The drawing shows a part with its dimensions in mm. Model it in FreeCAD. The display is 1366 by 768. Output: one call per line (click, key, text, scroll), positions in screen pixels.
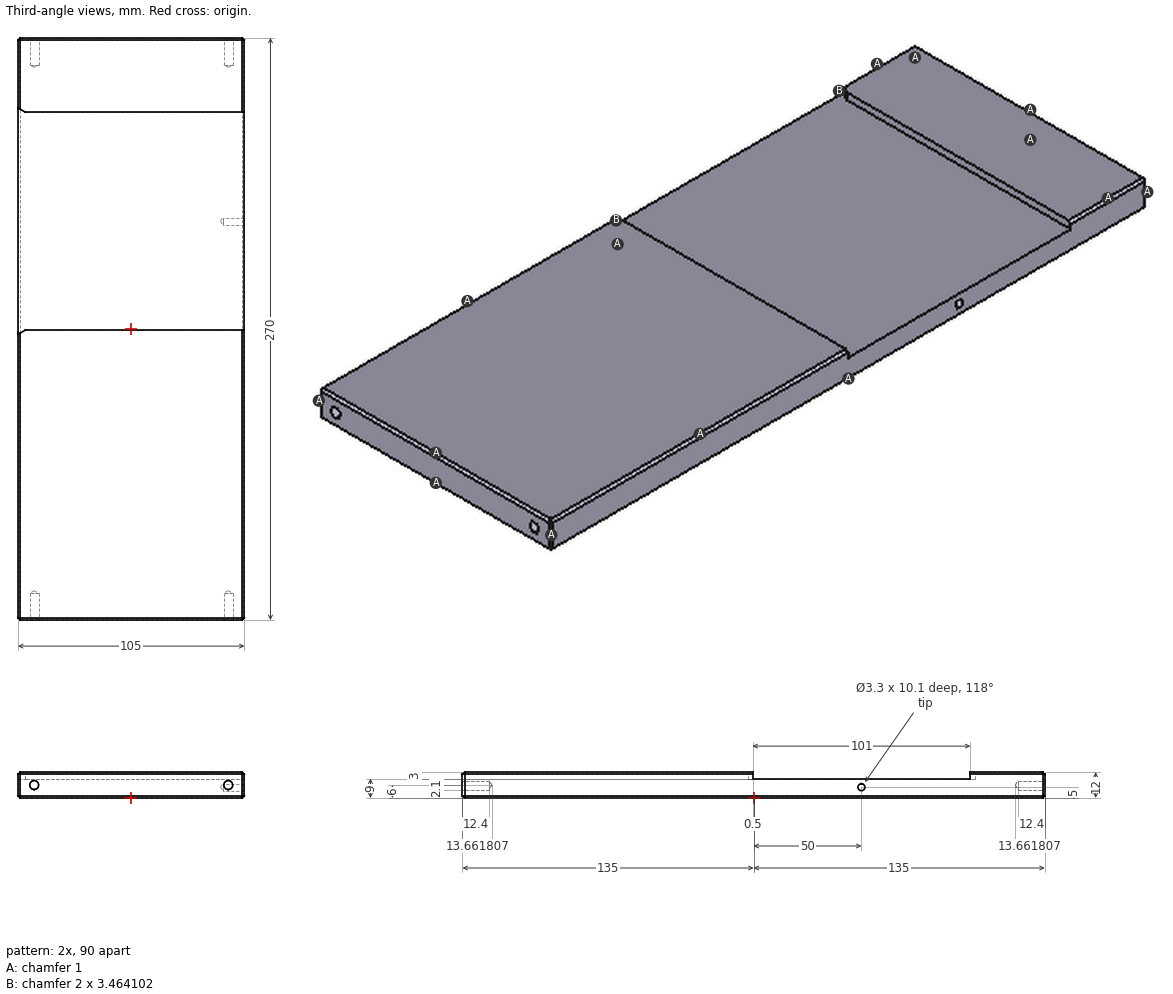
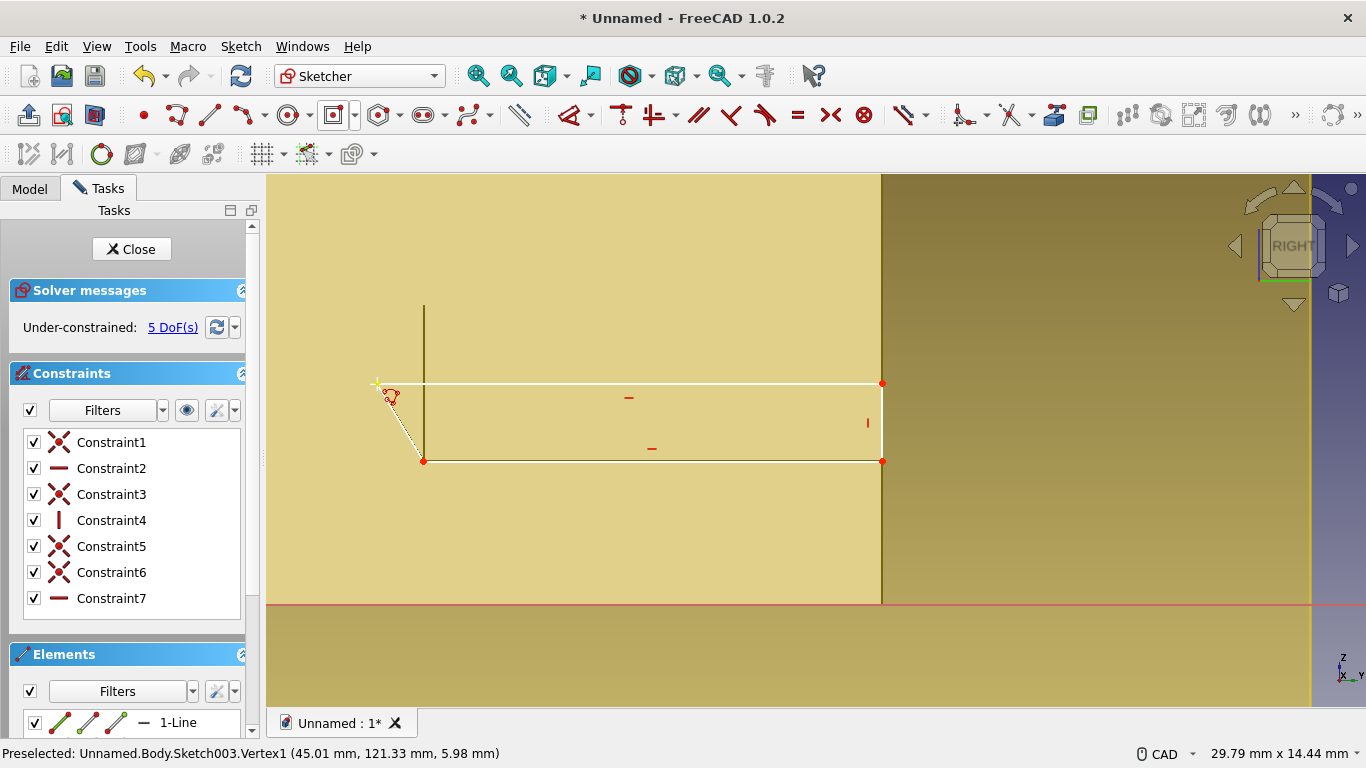
click(210, 116)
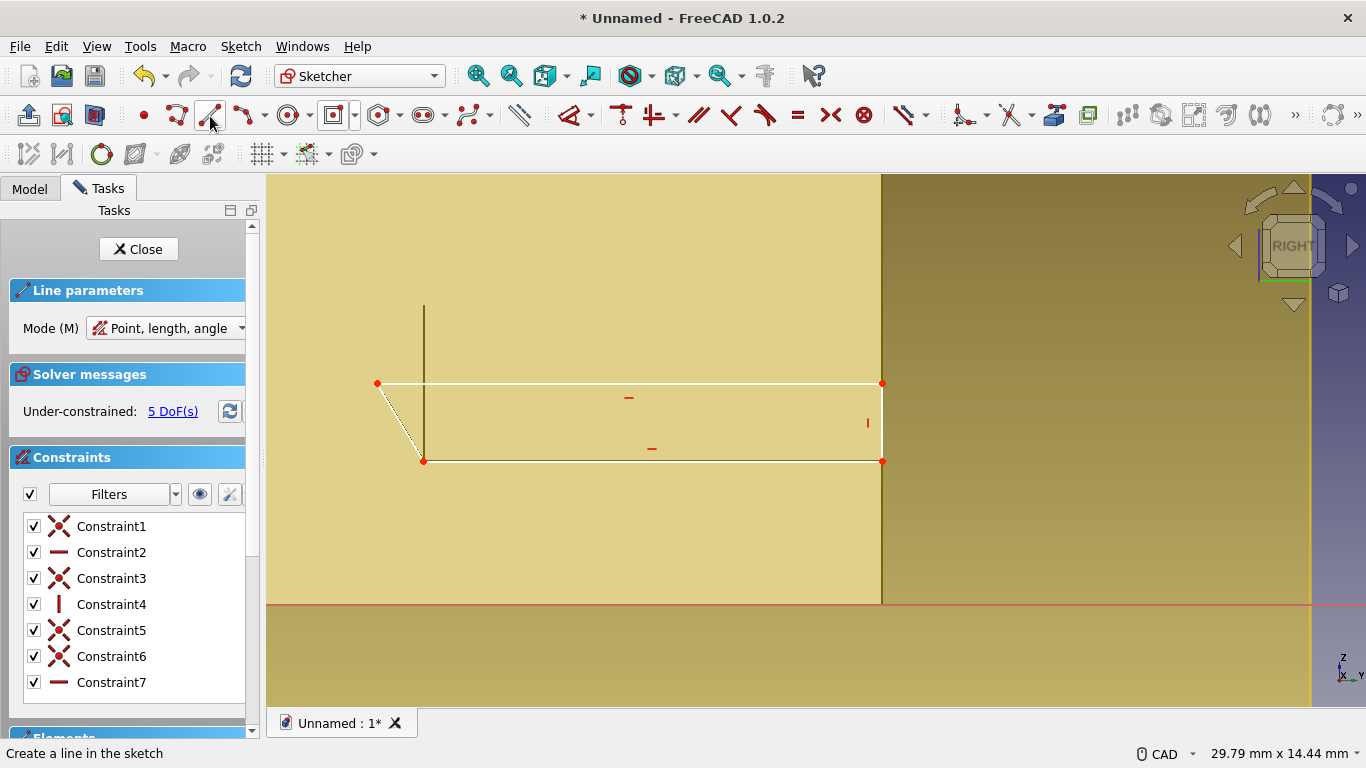
click(932, 383)
click(1083, 383)
key(Escape)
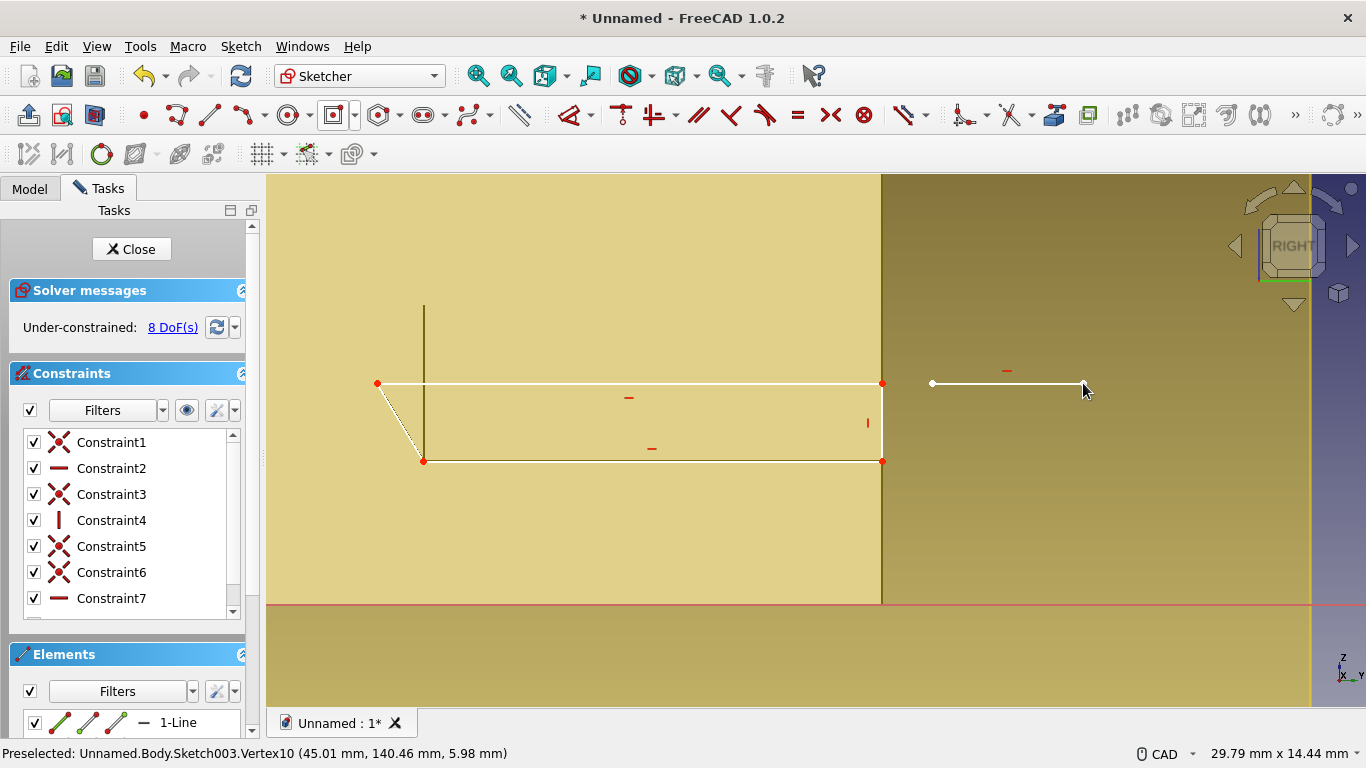
click(977, 384)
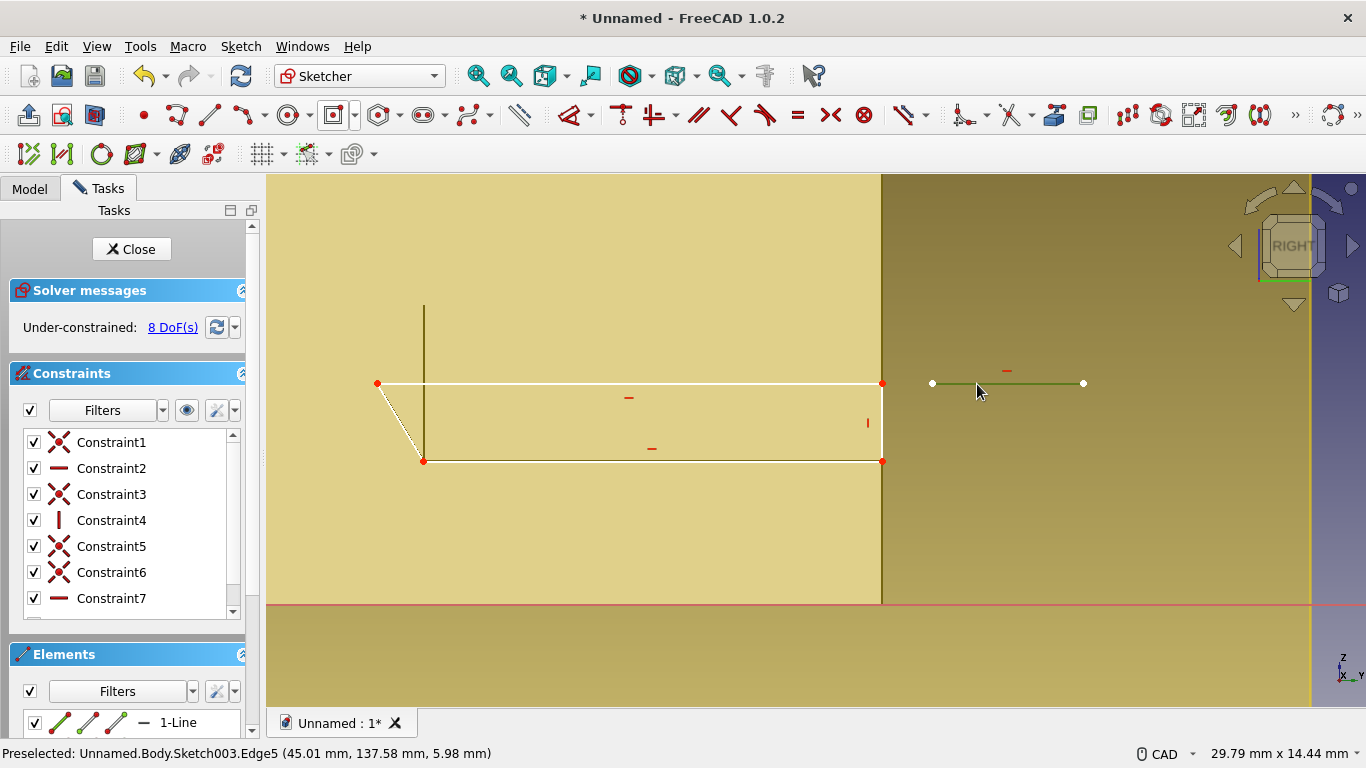
click(520, 116)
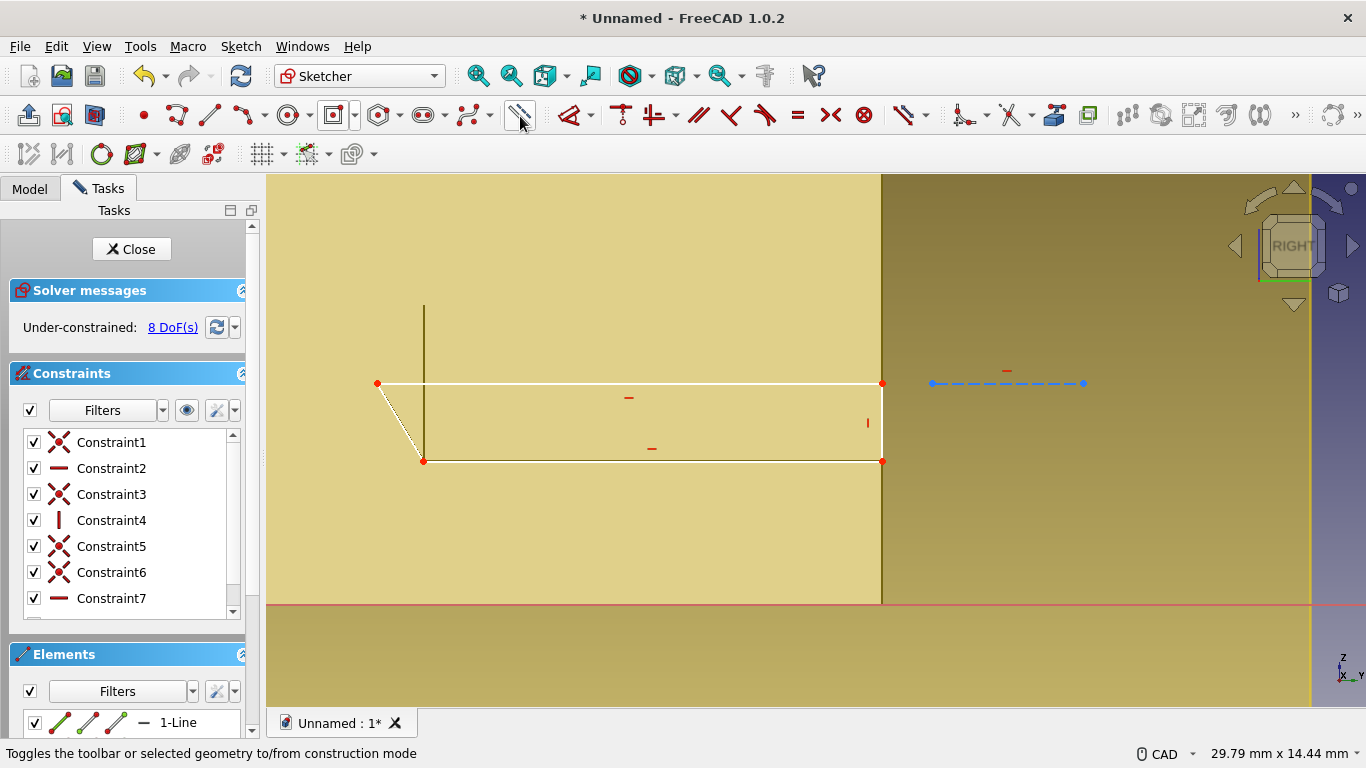
click(568, 116)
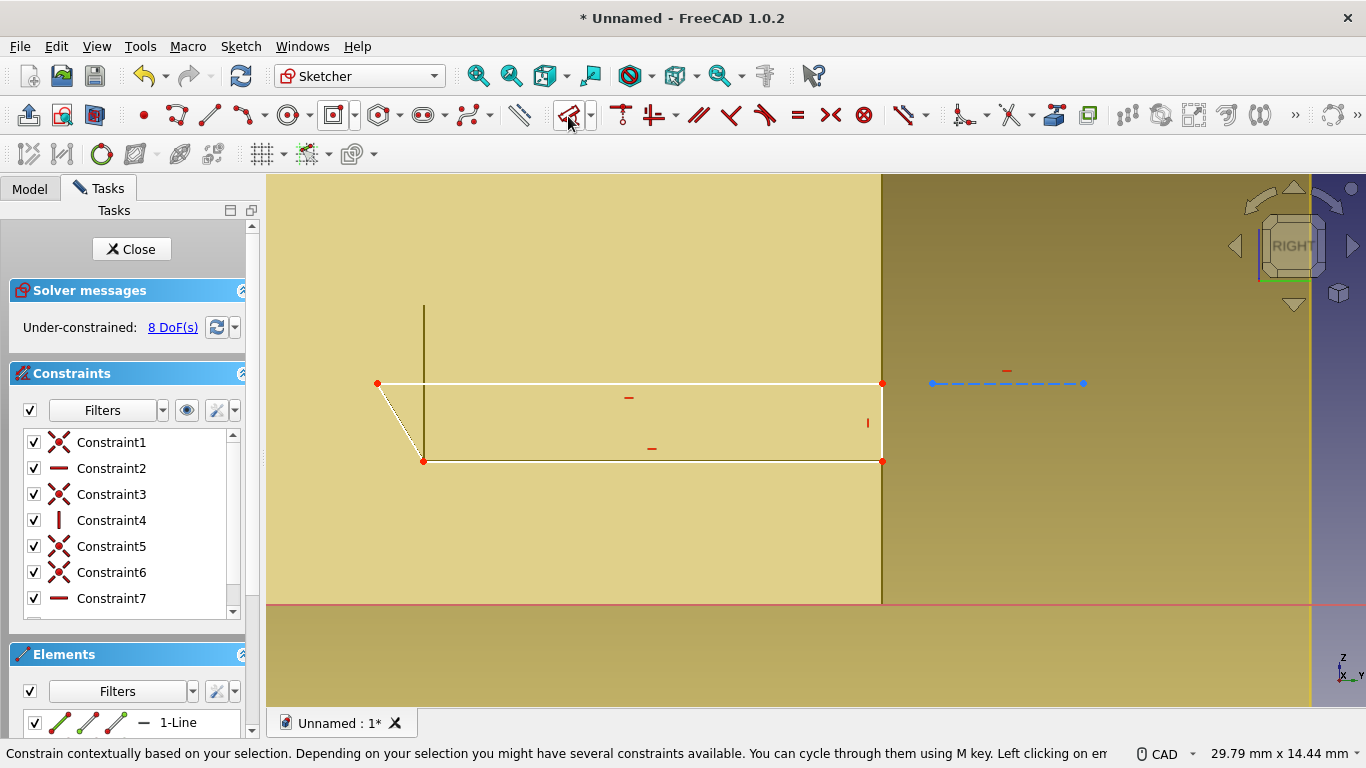
click(377, 384)
click(411, 494)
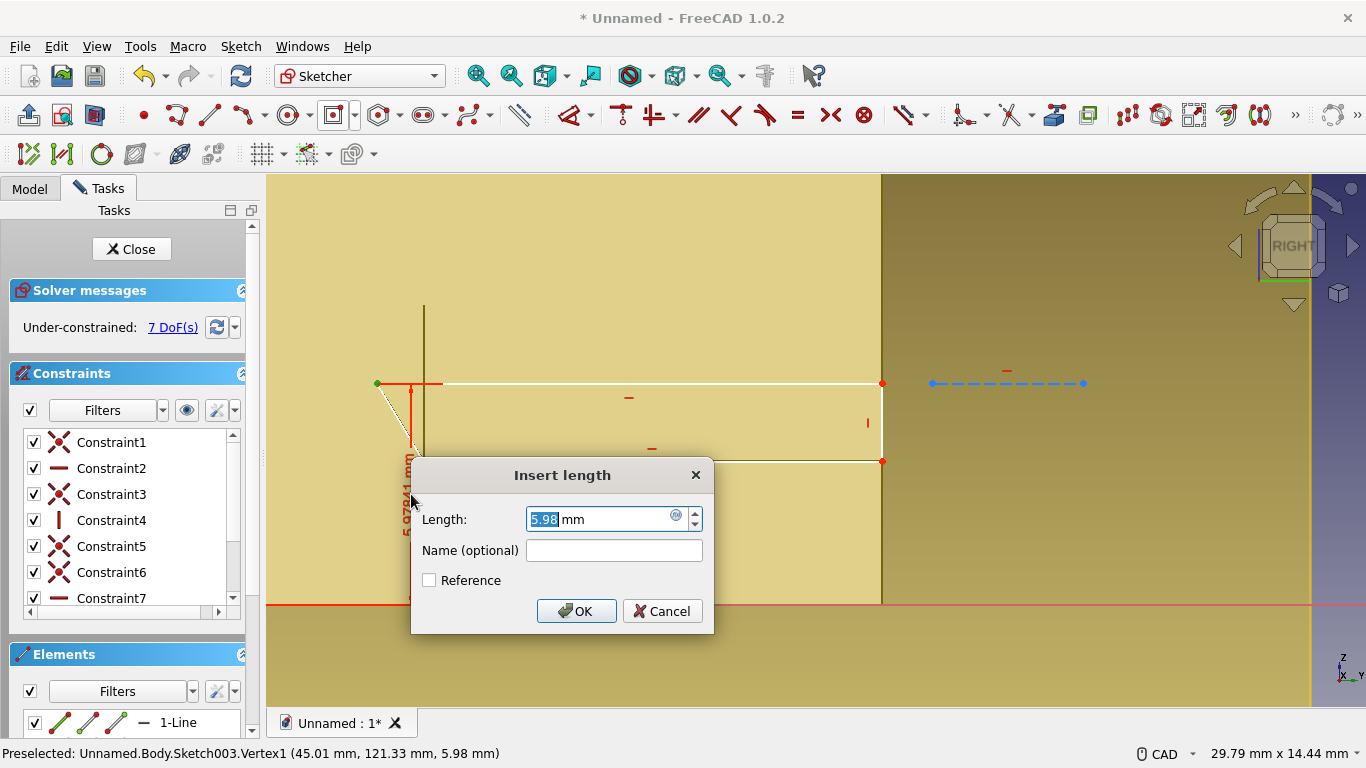
text(6)
key(Return)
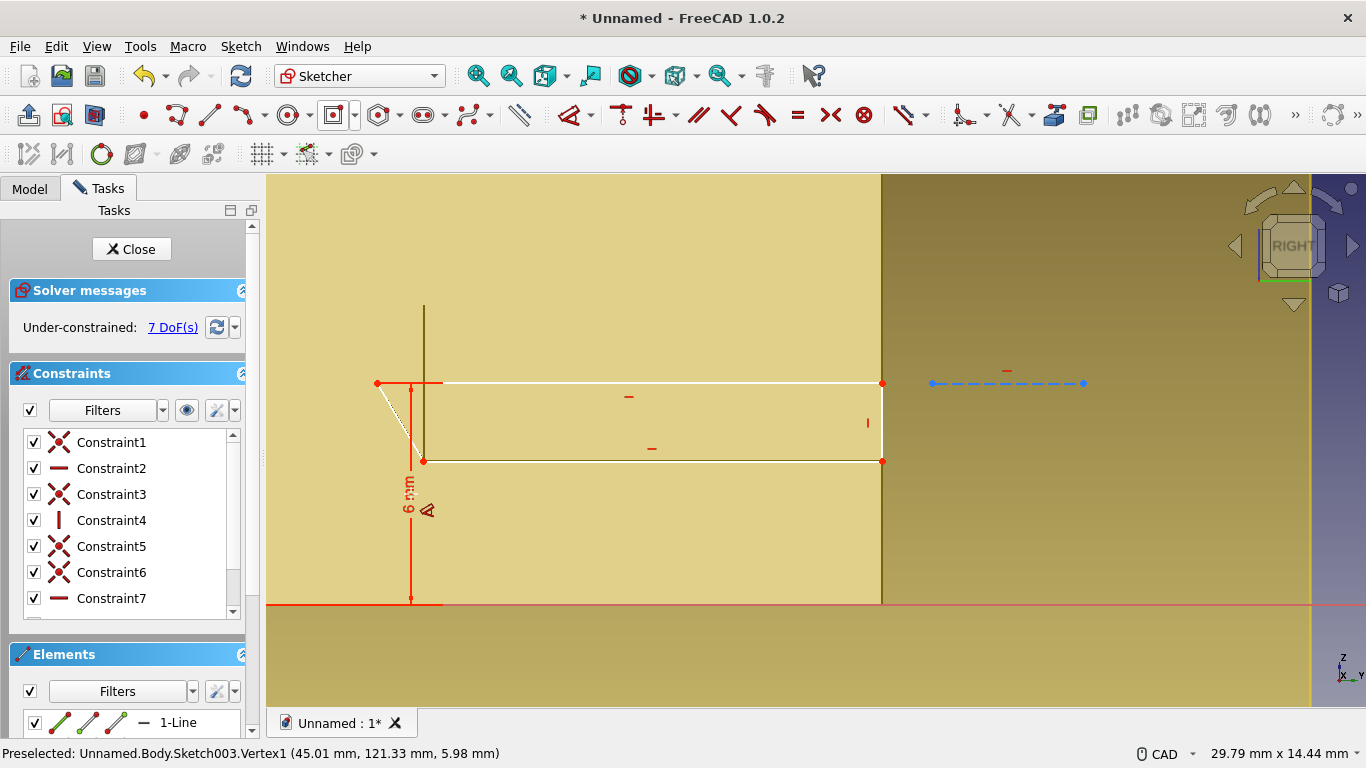
click(932, 384)
click(966, 494)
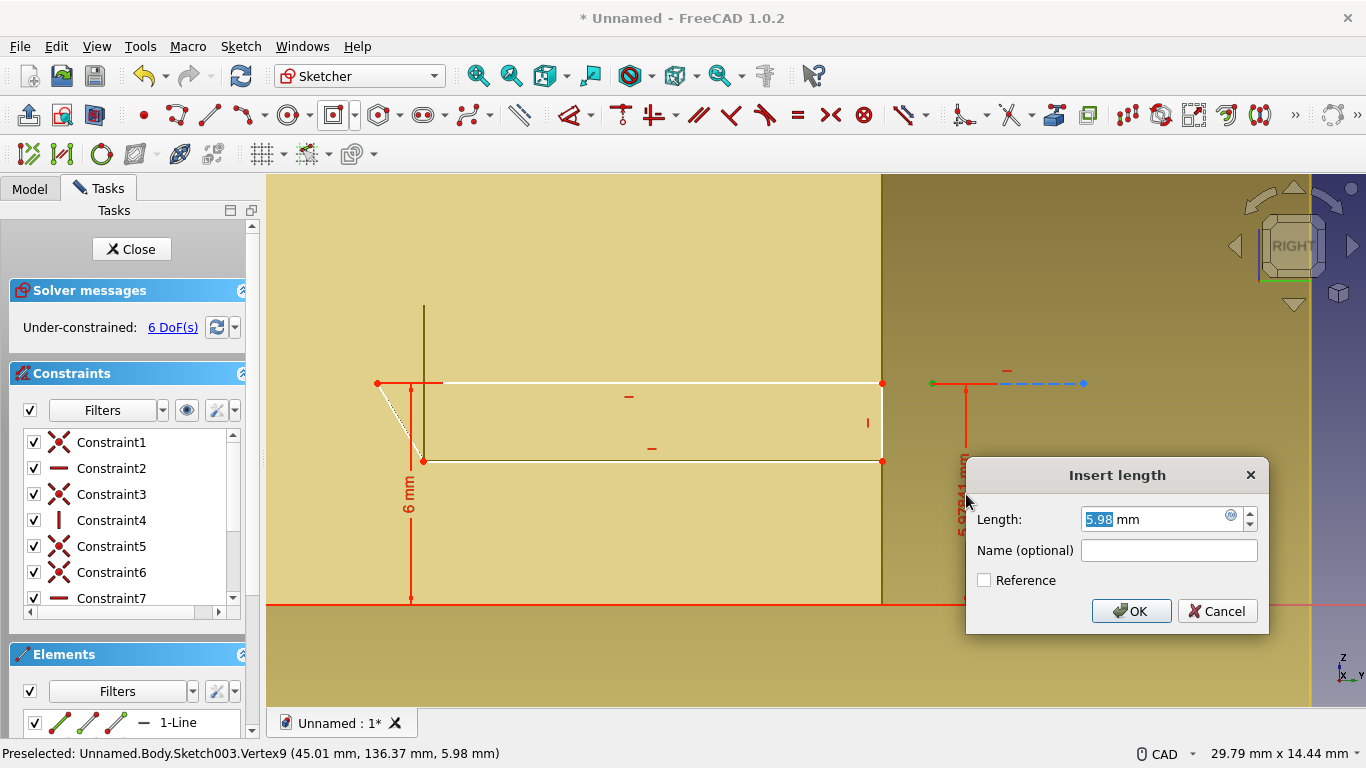
text(6)
key(Return)